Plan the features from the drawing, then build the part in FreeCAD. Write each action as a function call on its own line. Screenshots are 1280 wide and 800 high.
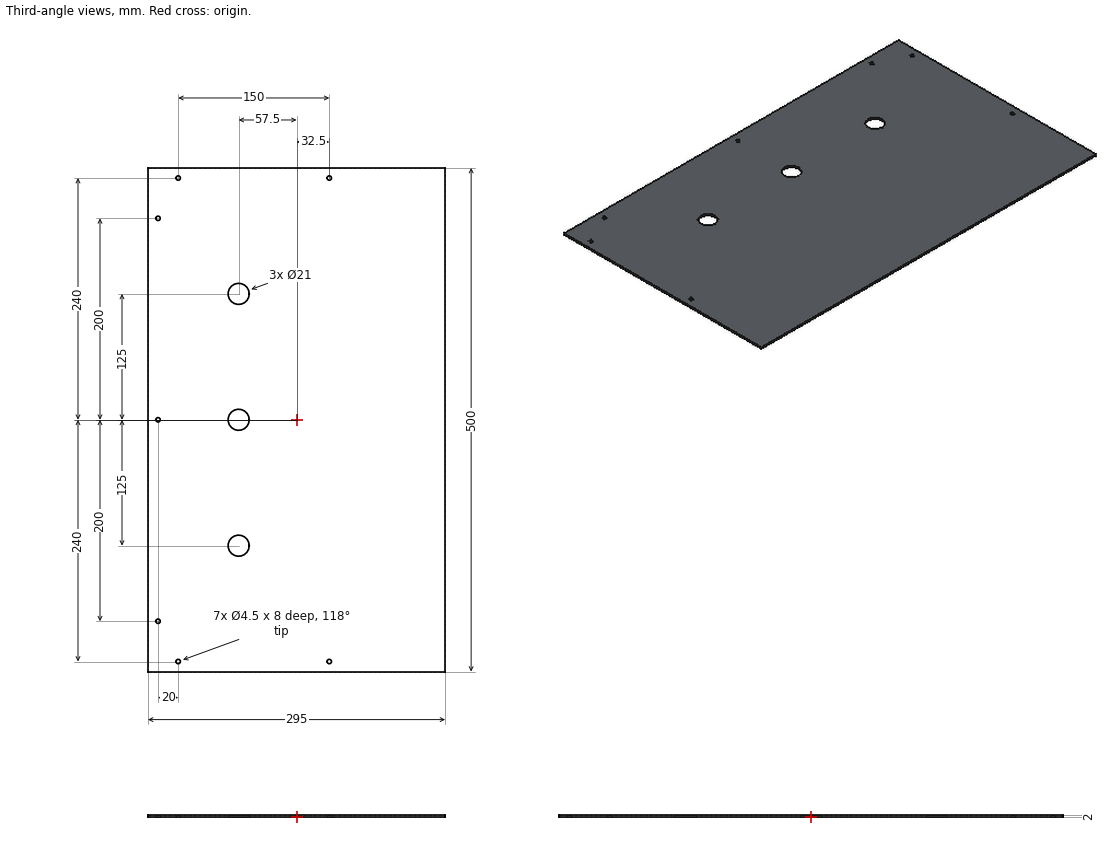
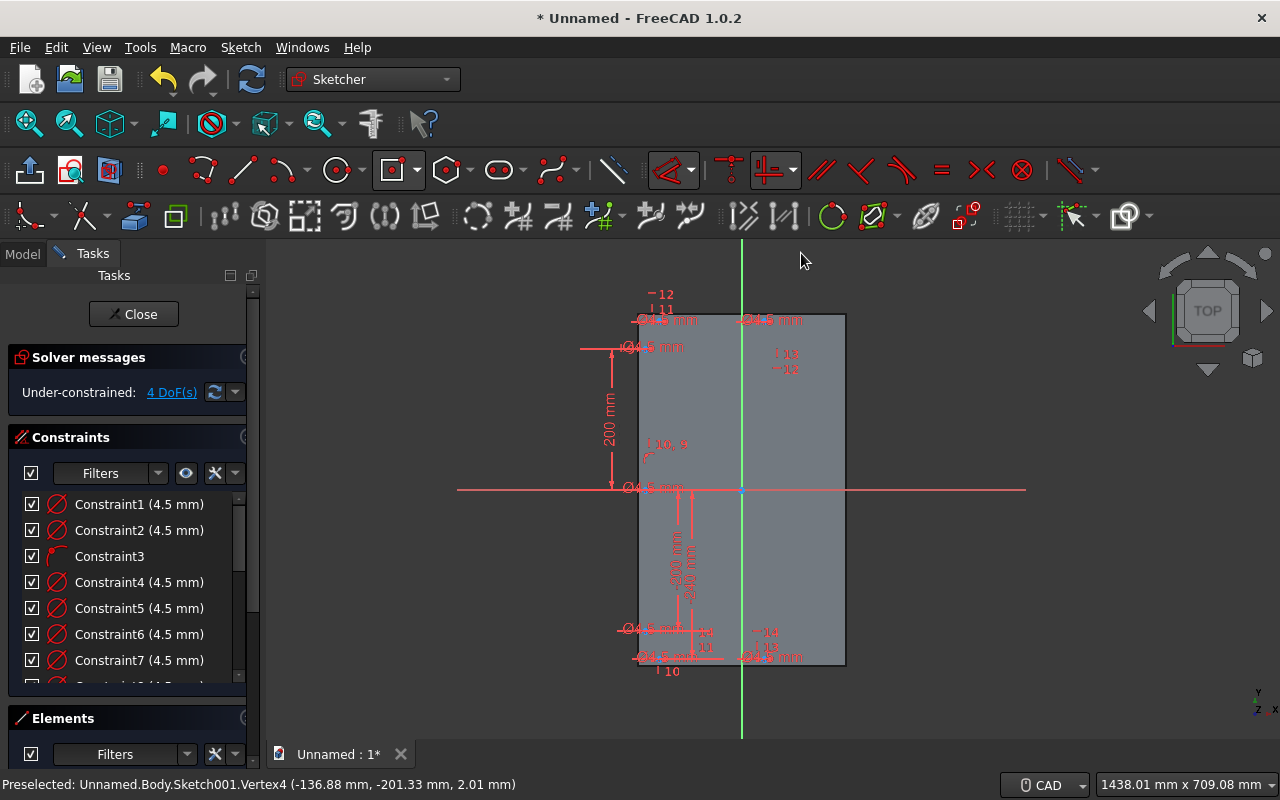
click(659, 322)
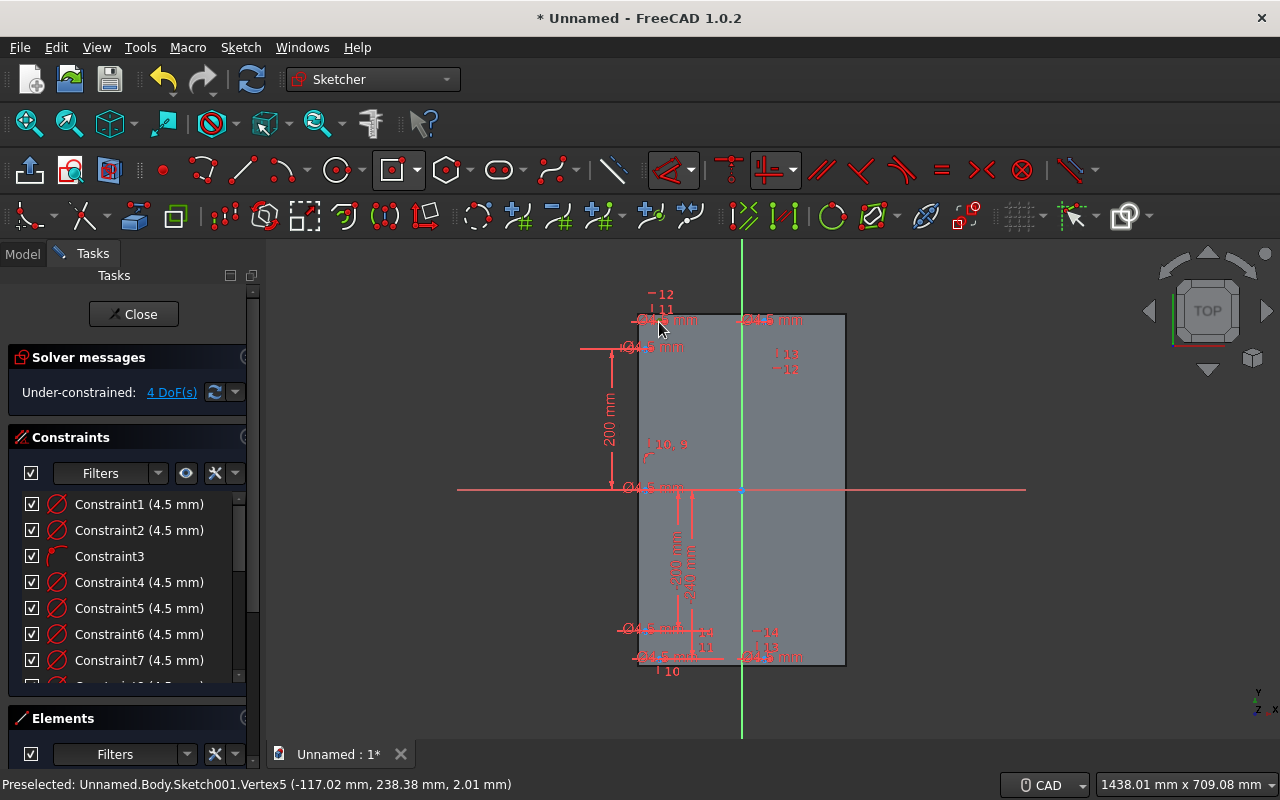
click(694, 170)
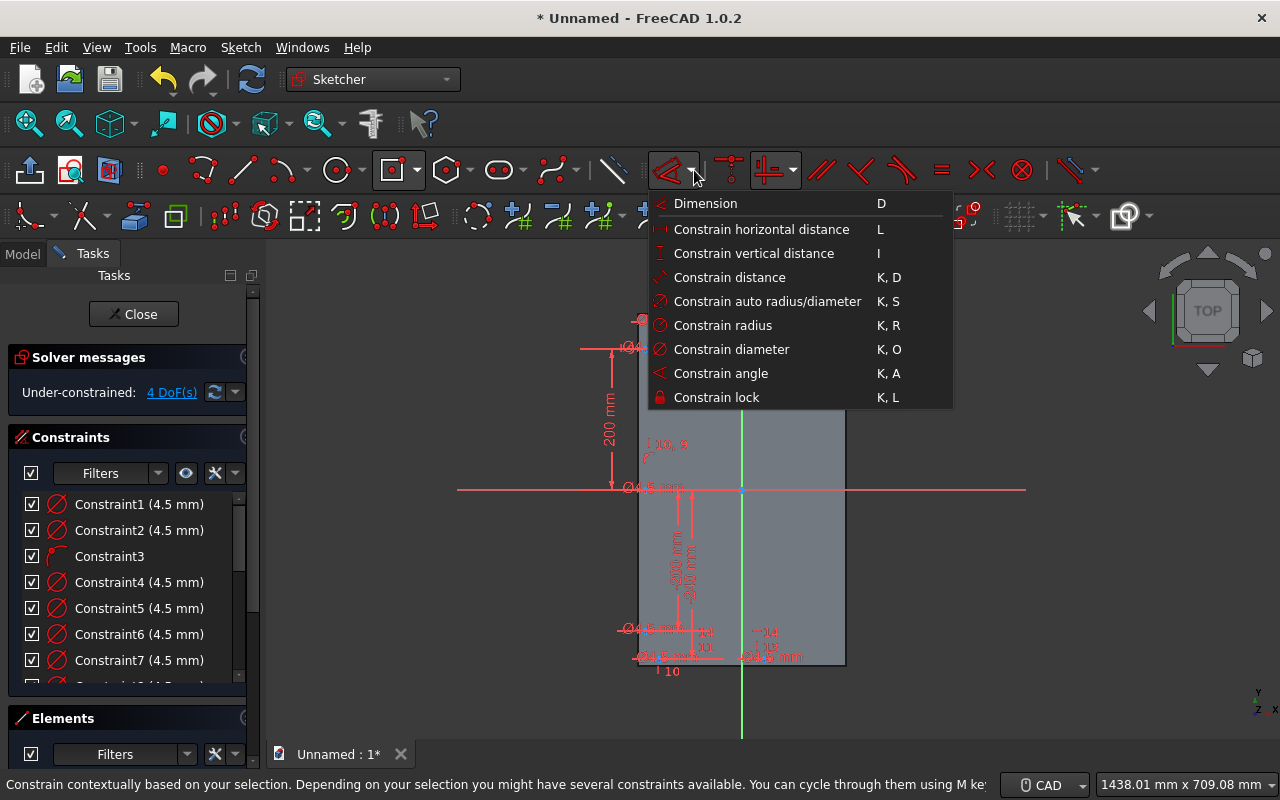
click(801, 253)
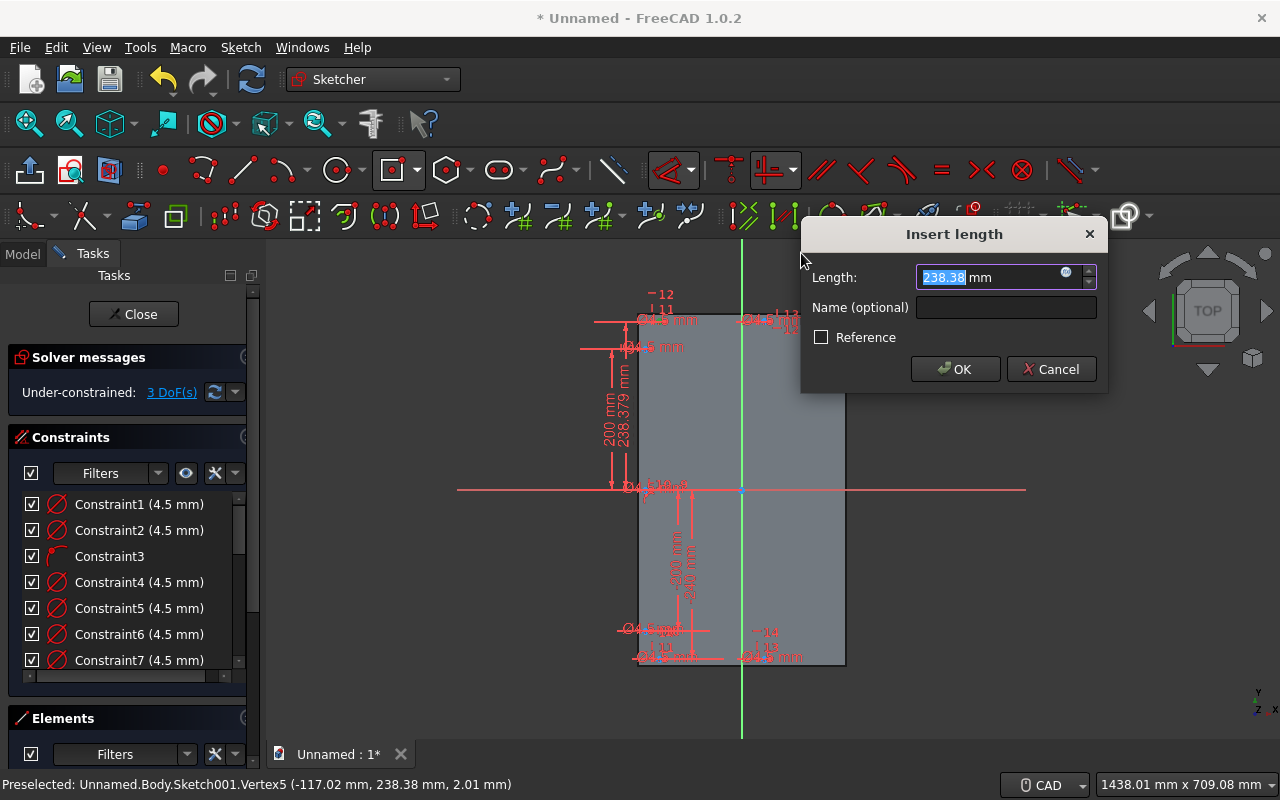
text(240)
key(Return)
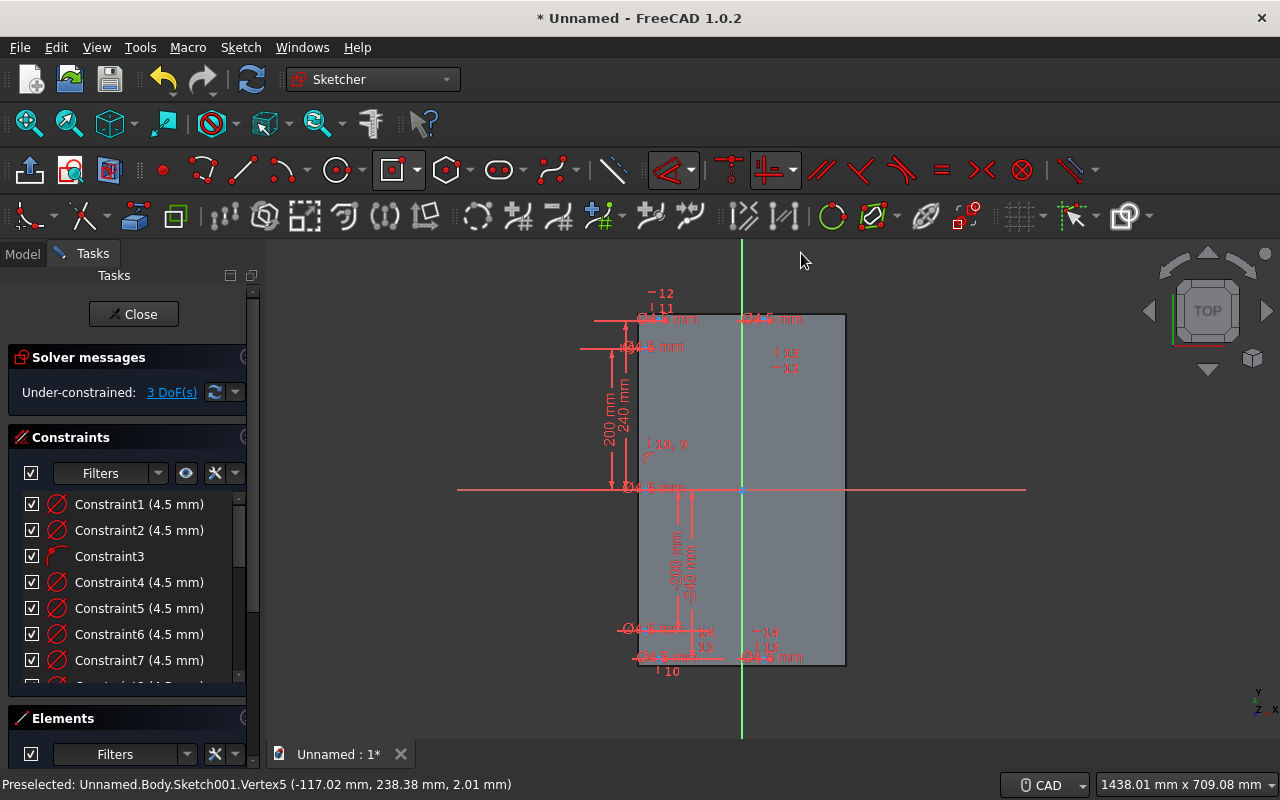
scroll(659, 659, up, 6)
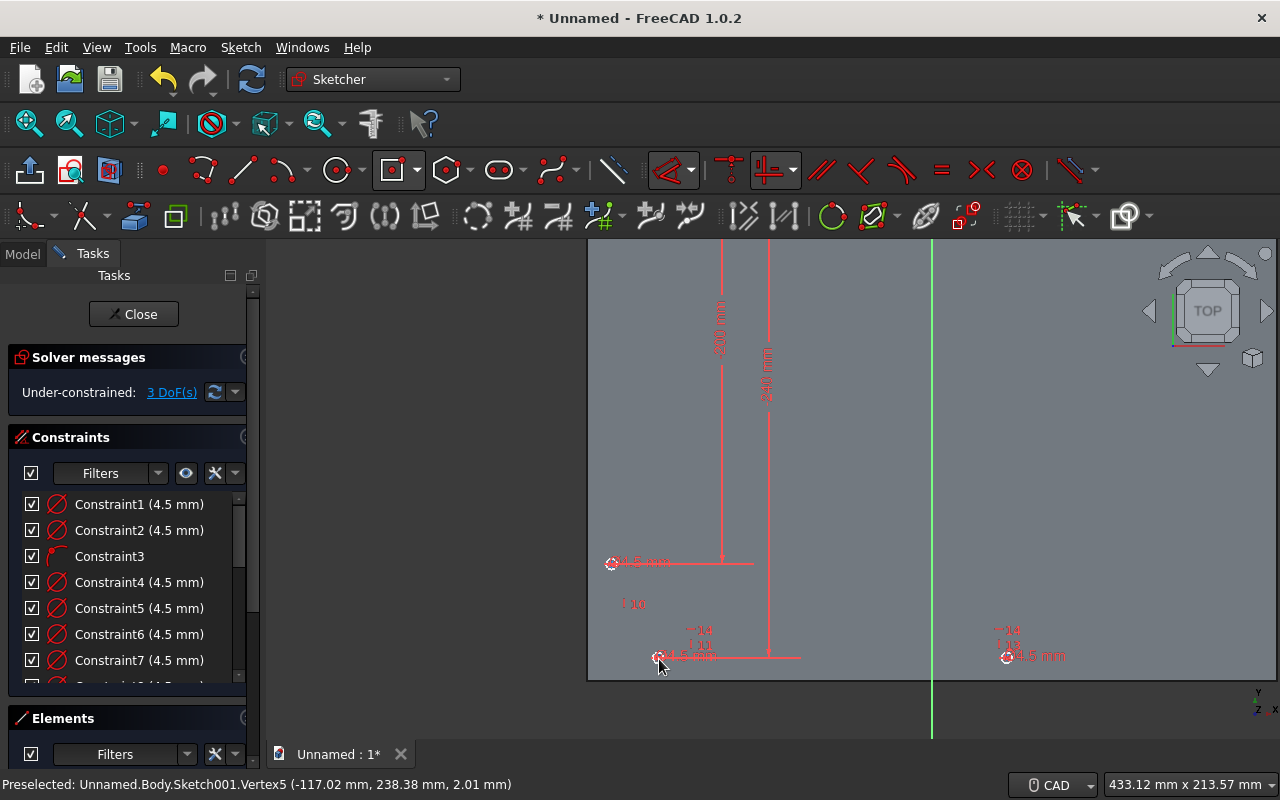
click(658, 658)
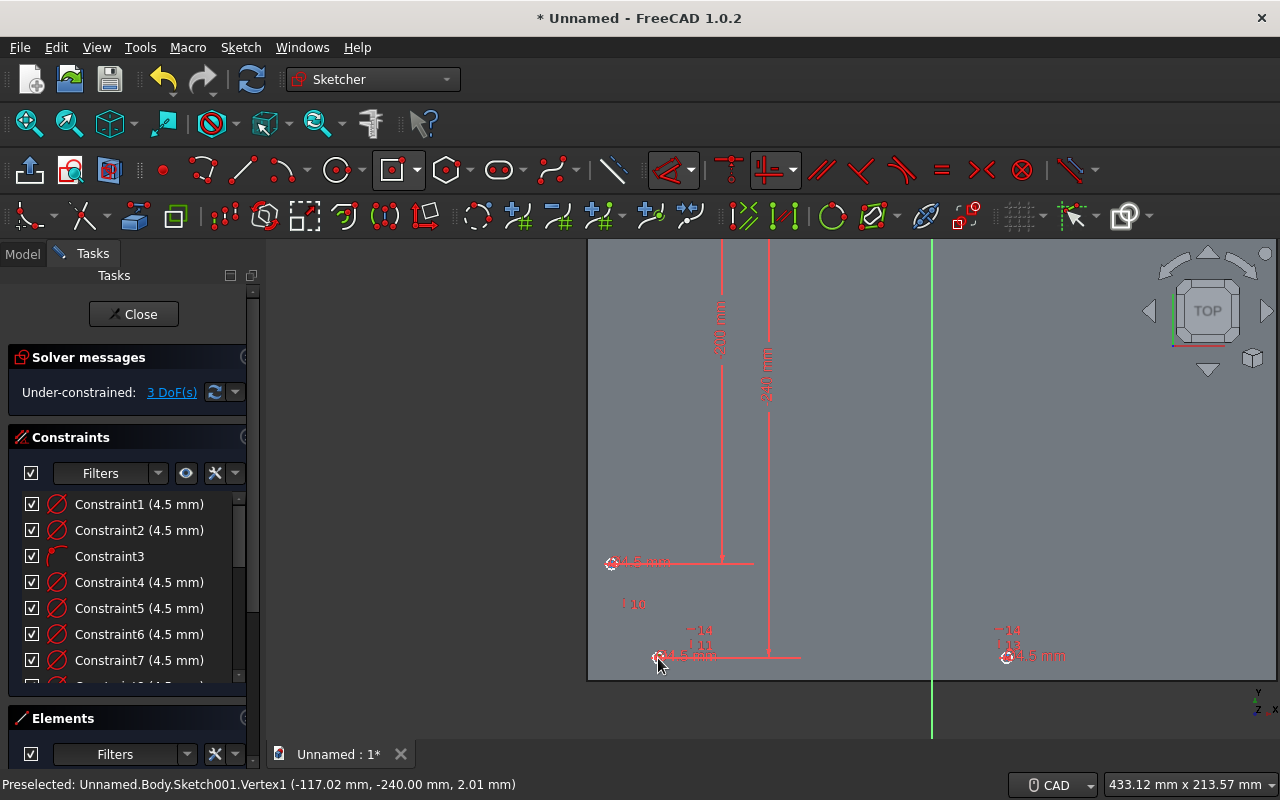
scroll(659, 658, down, 6)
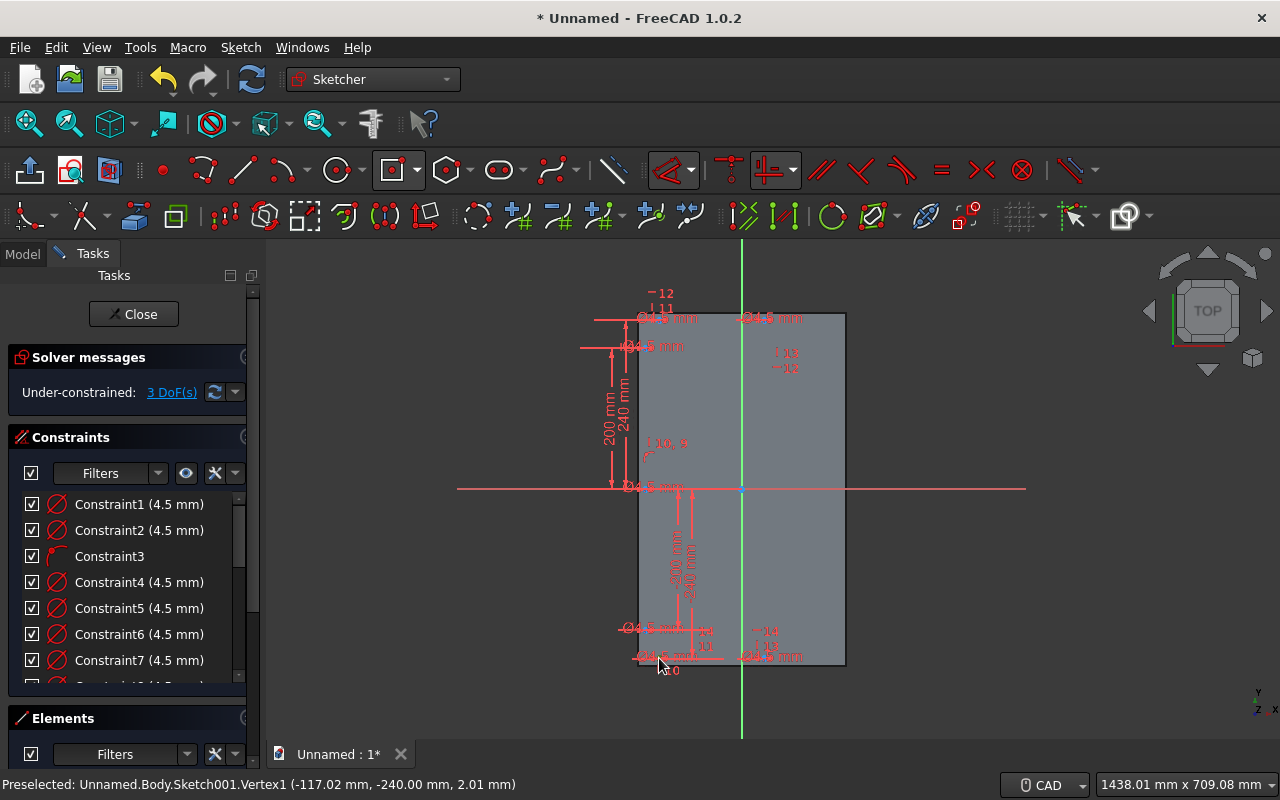
scroll(645, 489, up, 6)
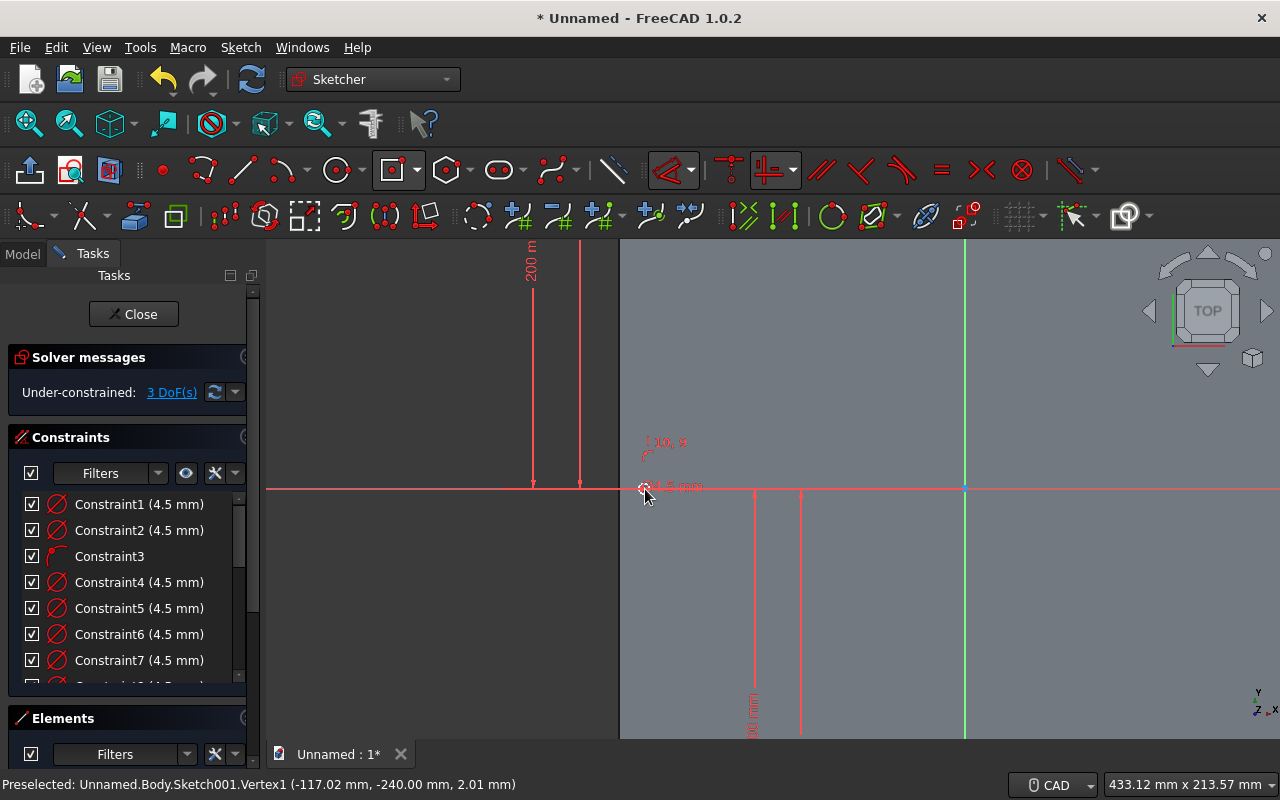
click(644, 489)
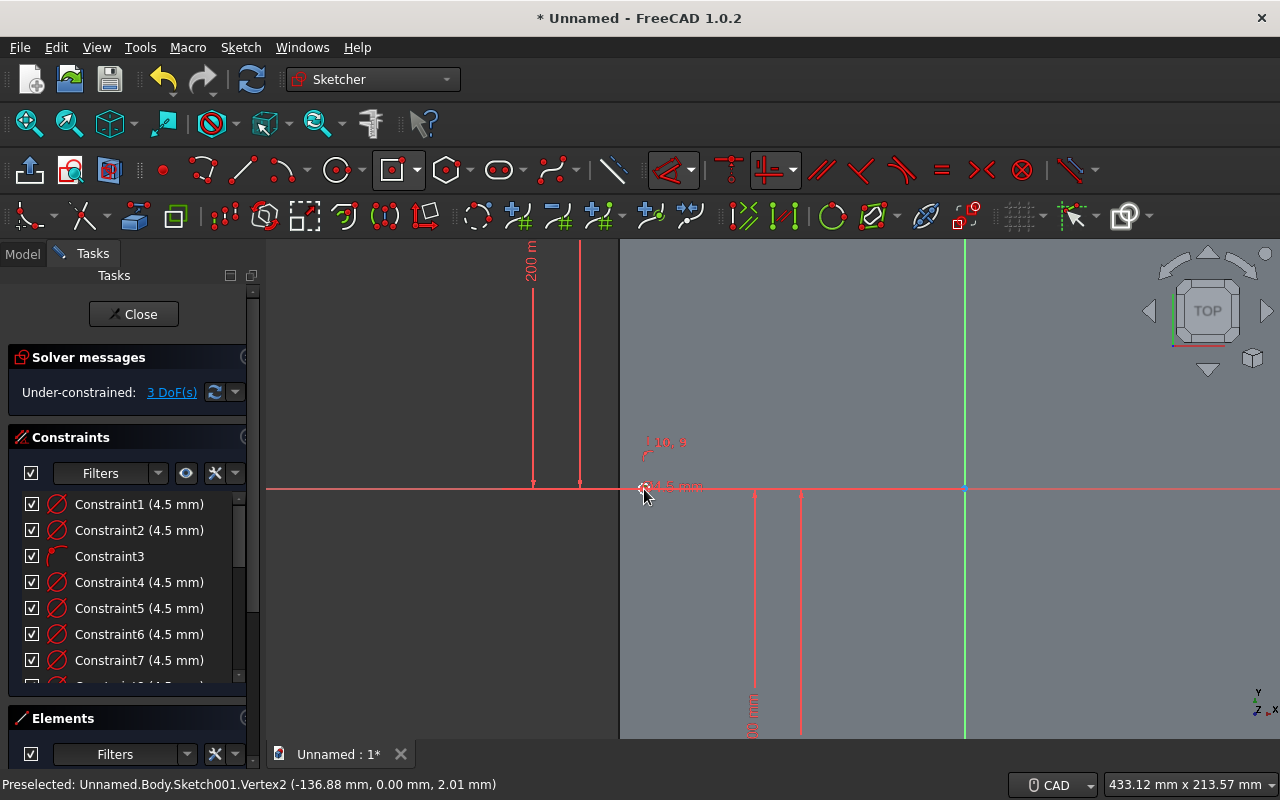
click(694, 170)